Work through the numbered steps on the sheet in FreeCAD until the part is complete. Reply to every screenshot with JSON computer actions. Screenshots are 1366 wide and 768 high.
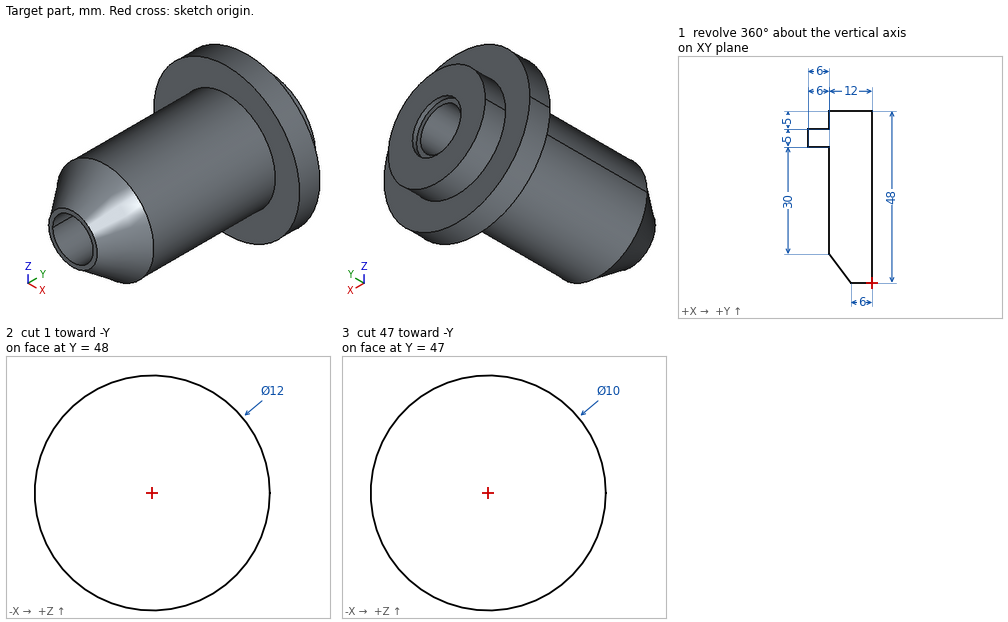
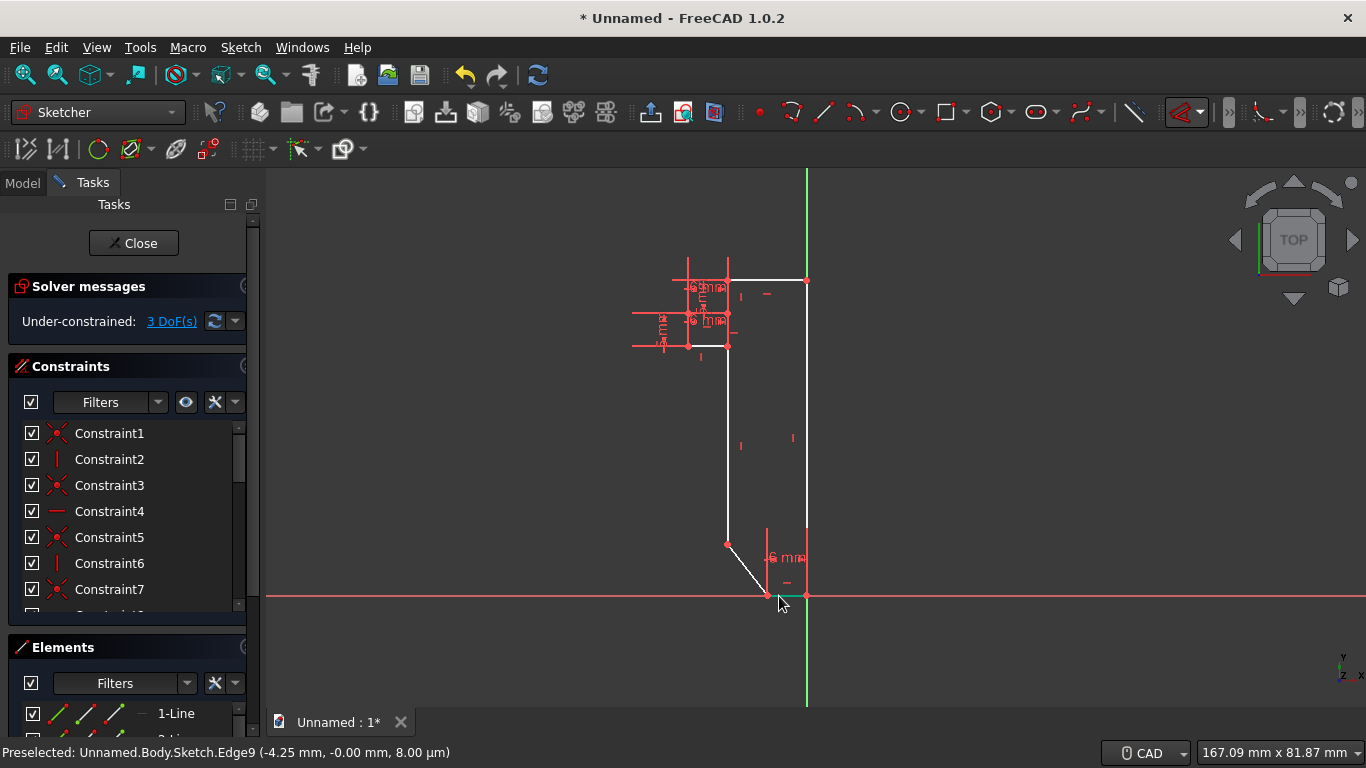
{"action": "left_click", "coordinate": [807, 501]}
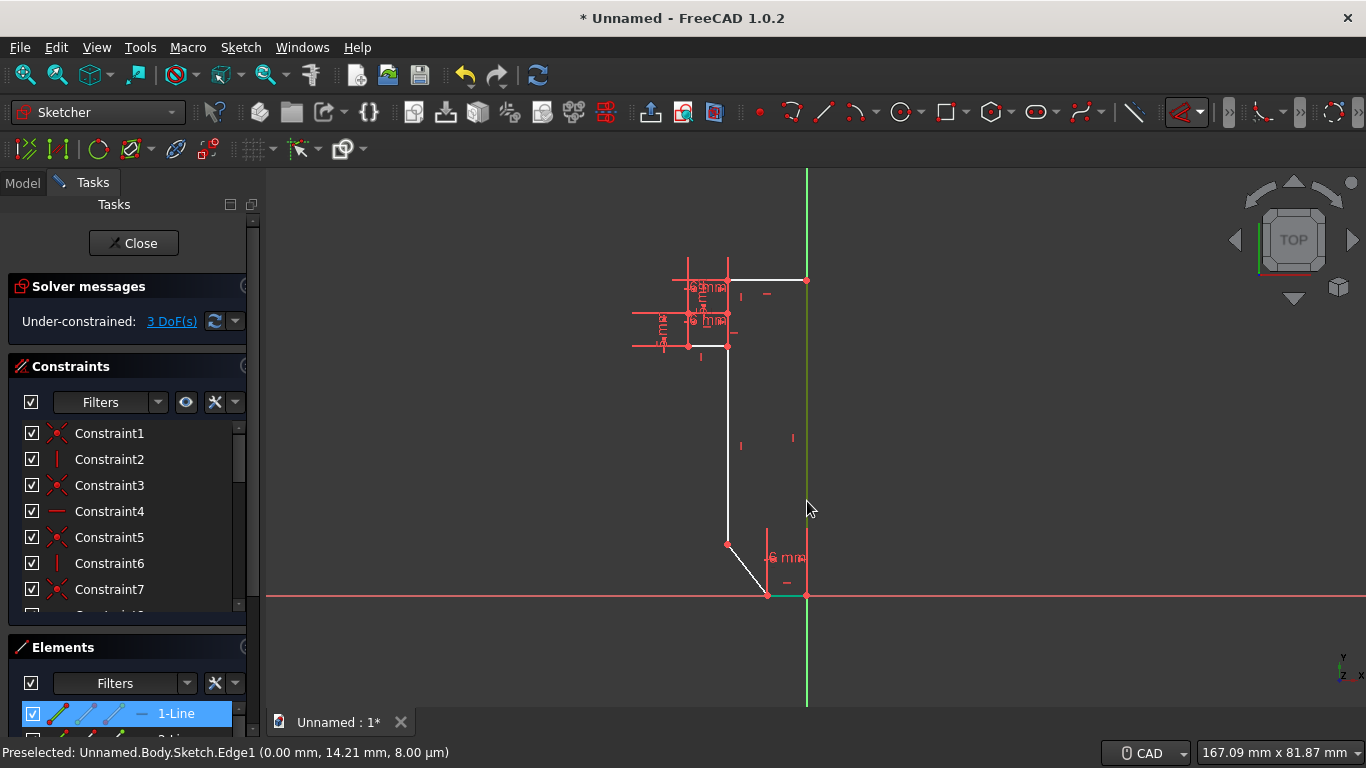
{"action": "key", "text": "i"}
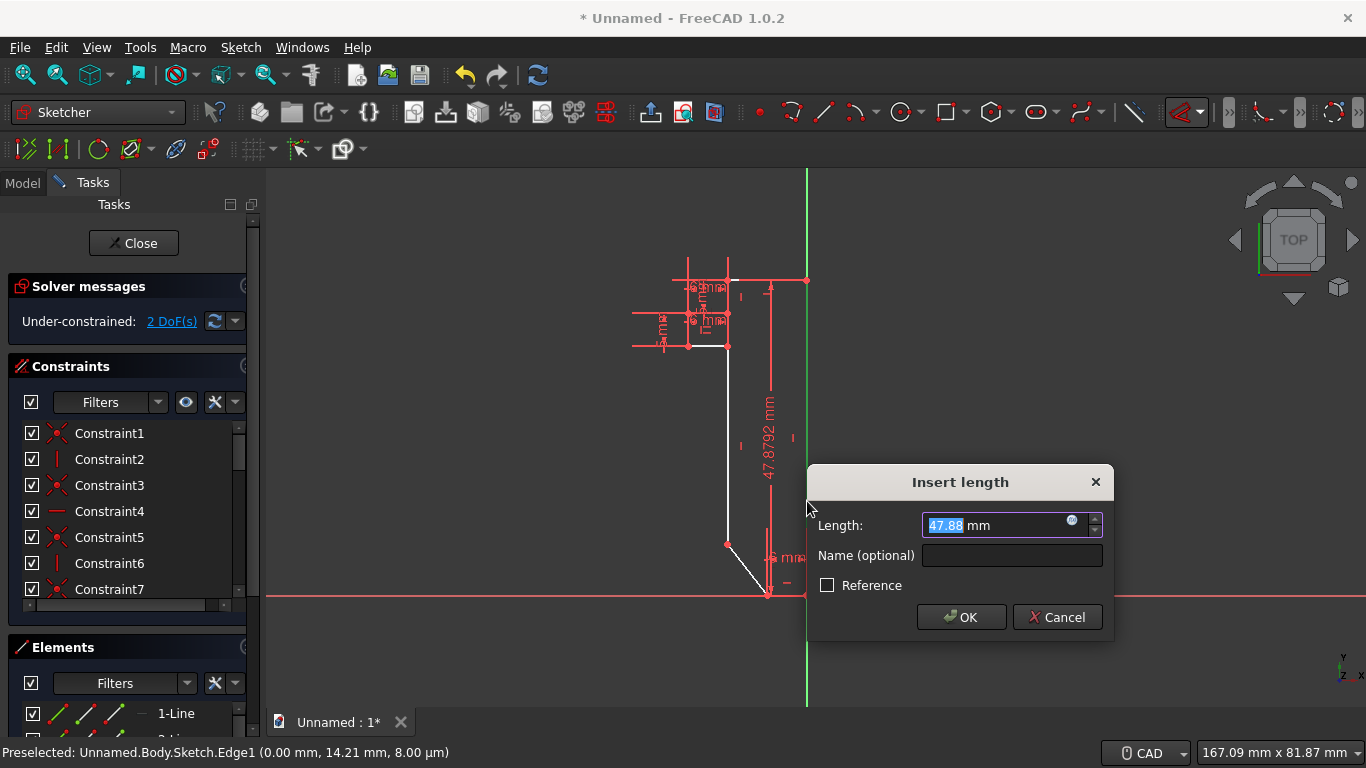
{"action": "type", "text": "48"}
{"action": "key", "text": "Return"}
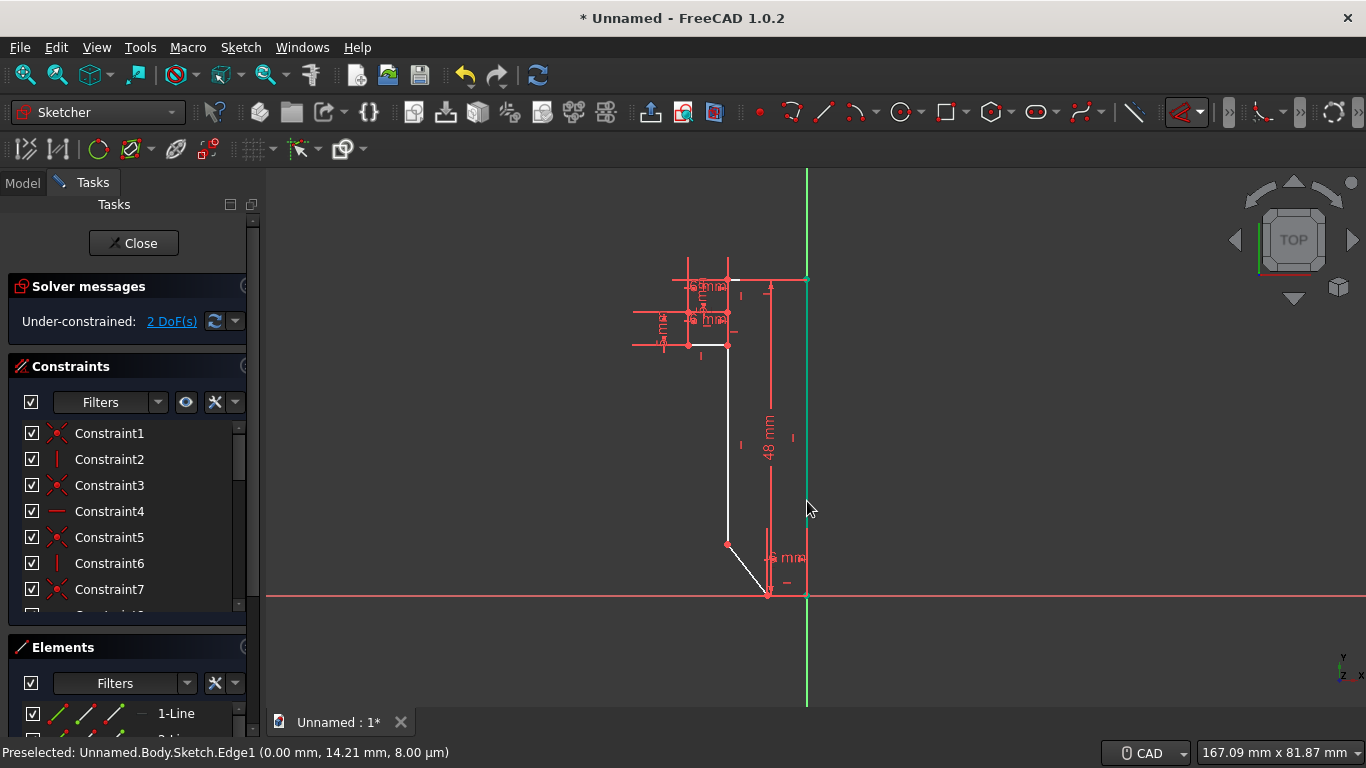
{"action": "left_click", "coordinate": [783, 280]}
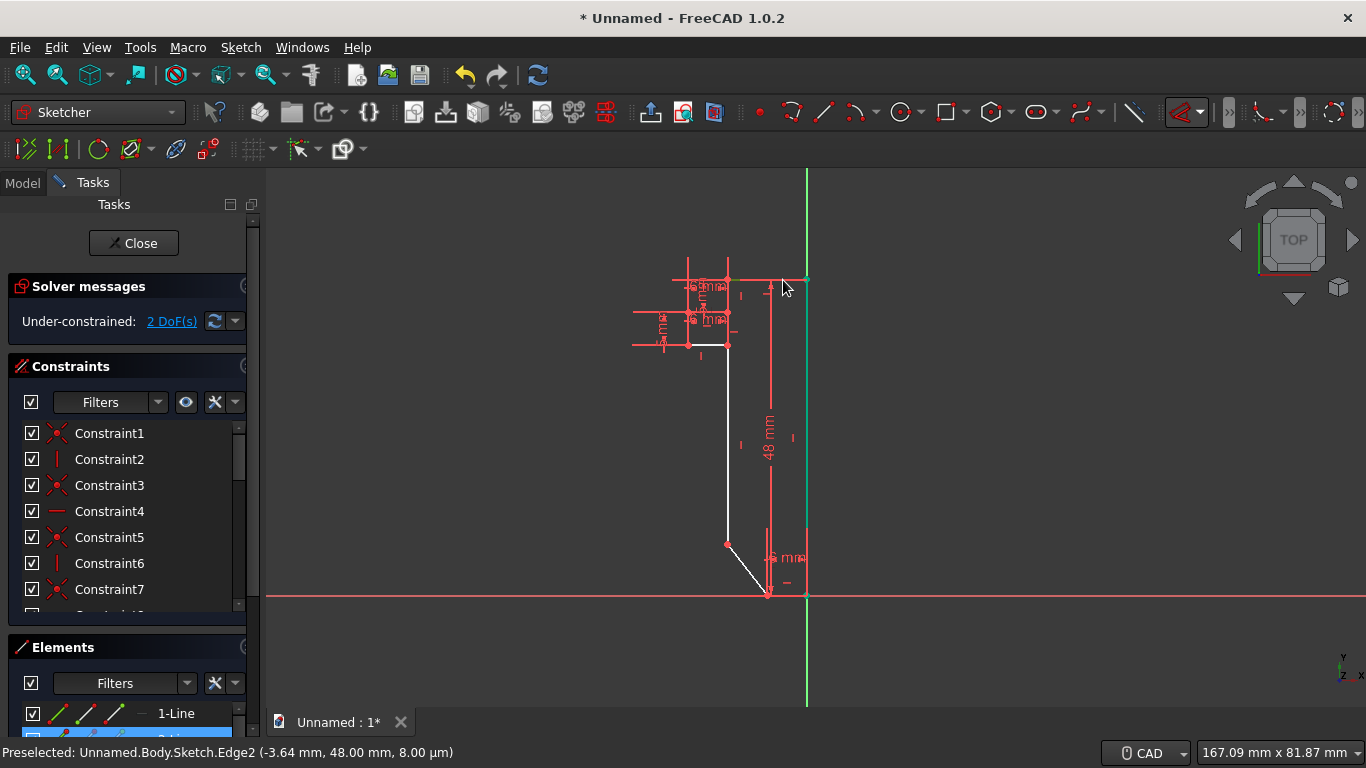
{"action": "left_click", "coordinate": [1202, 112]}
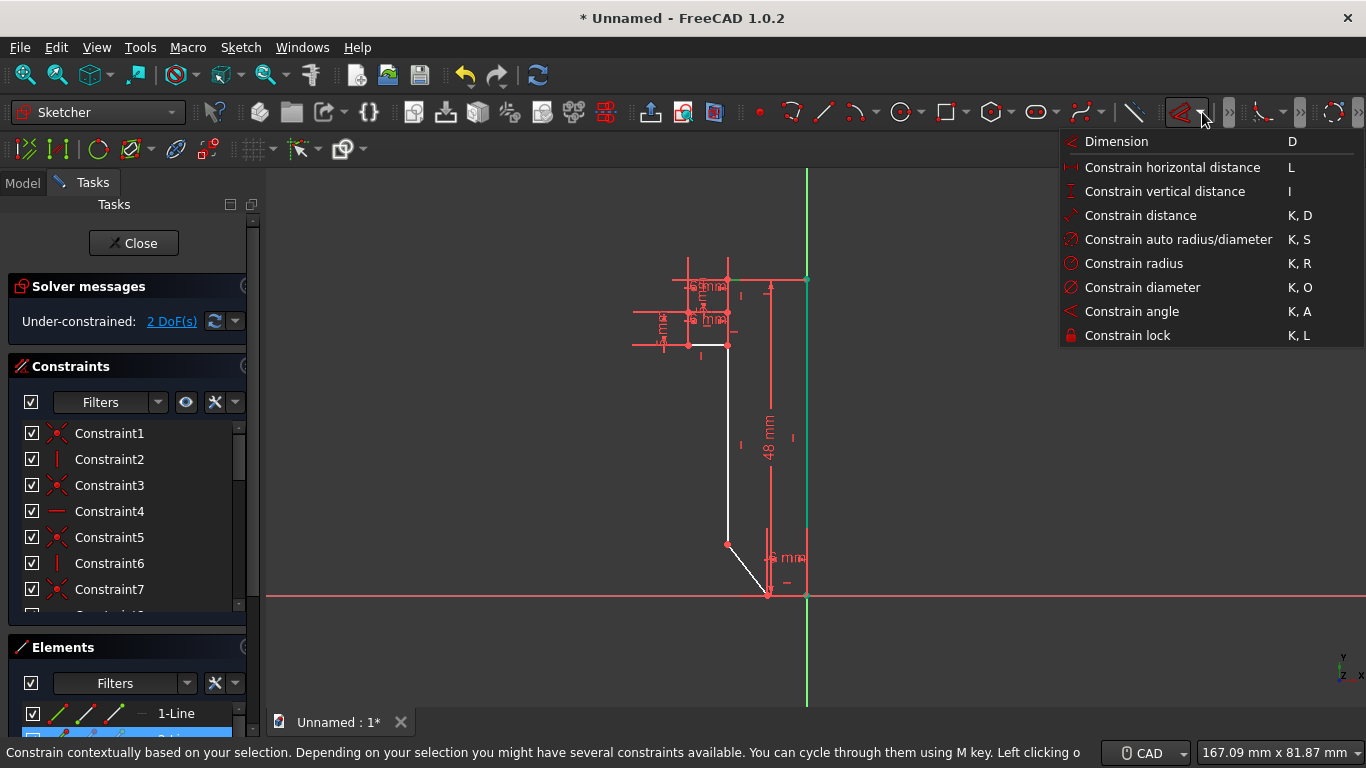
{"action": "left_click", "coordinate": [1212, 167]}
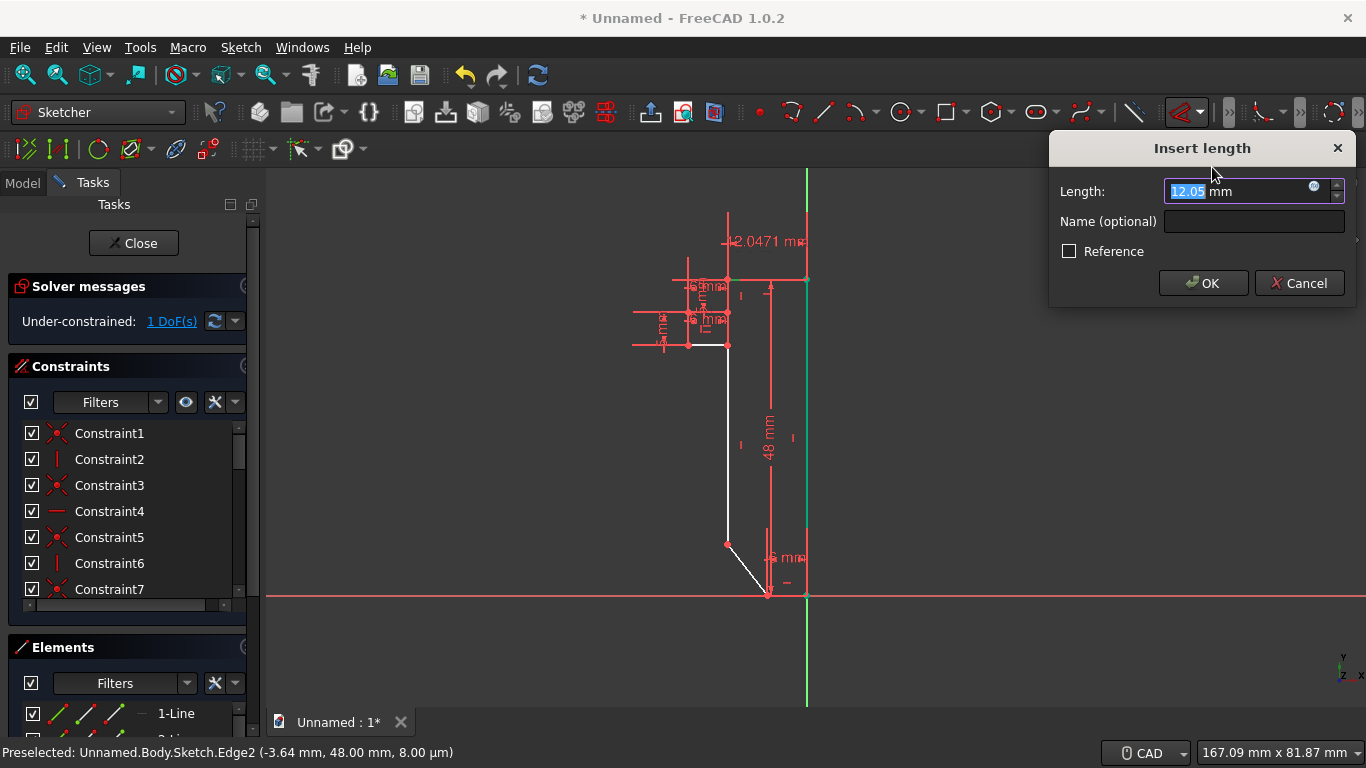
{"action": "type", "text": "12"}
{"action": "key", "text": "Return"}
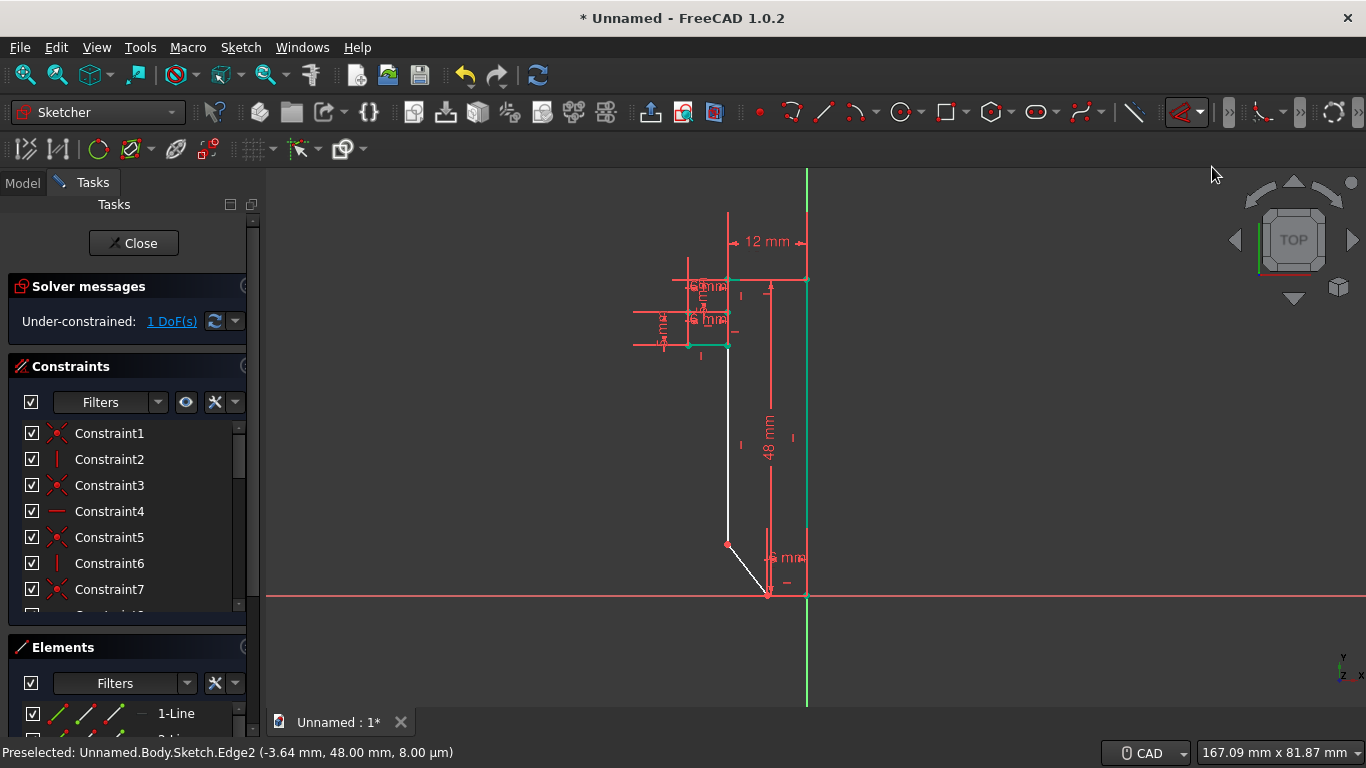
{"action": "left_click", "coordinate": [728, 405]}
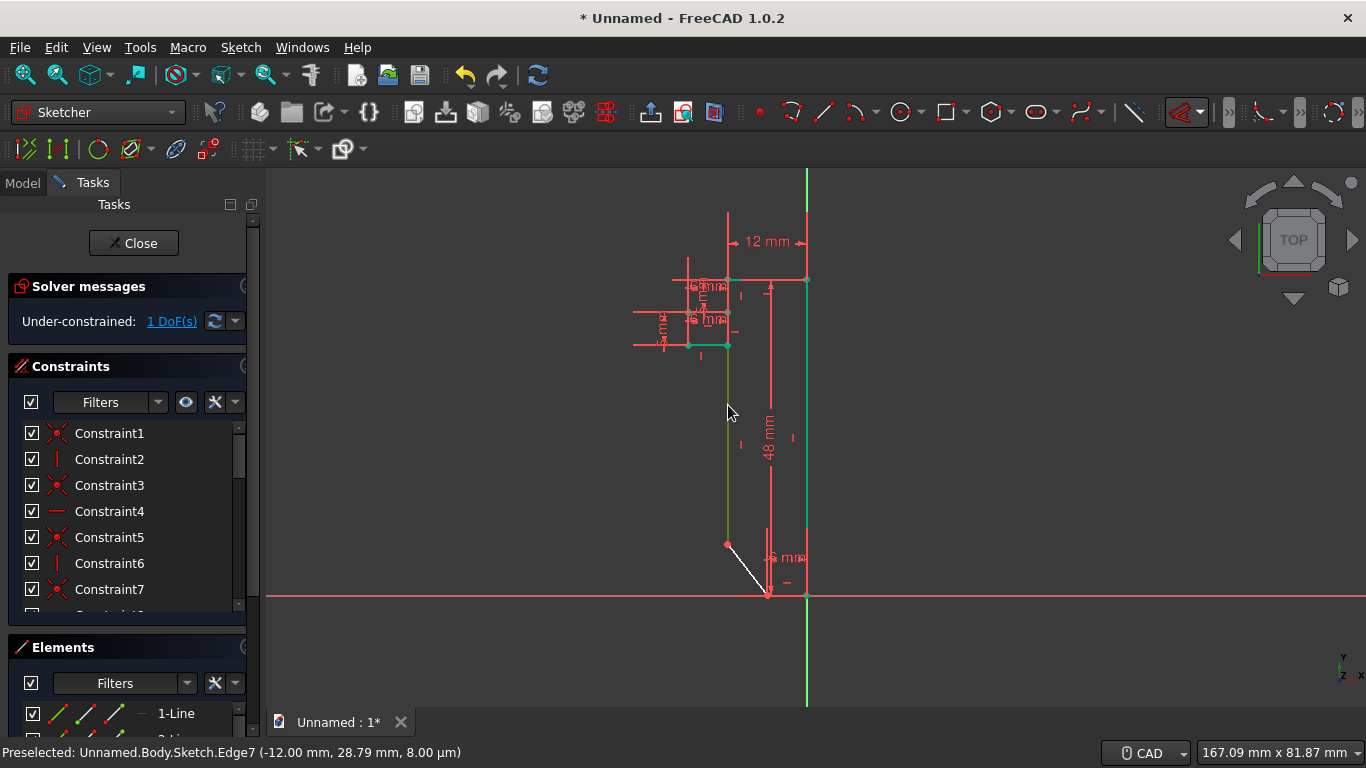
{"action": "left_click", "coordinate": [1202, 112]}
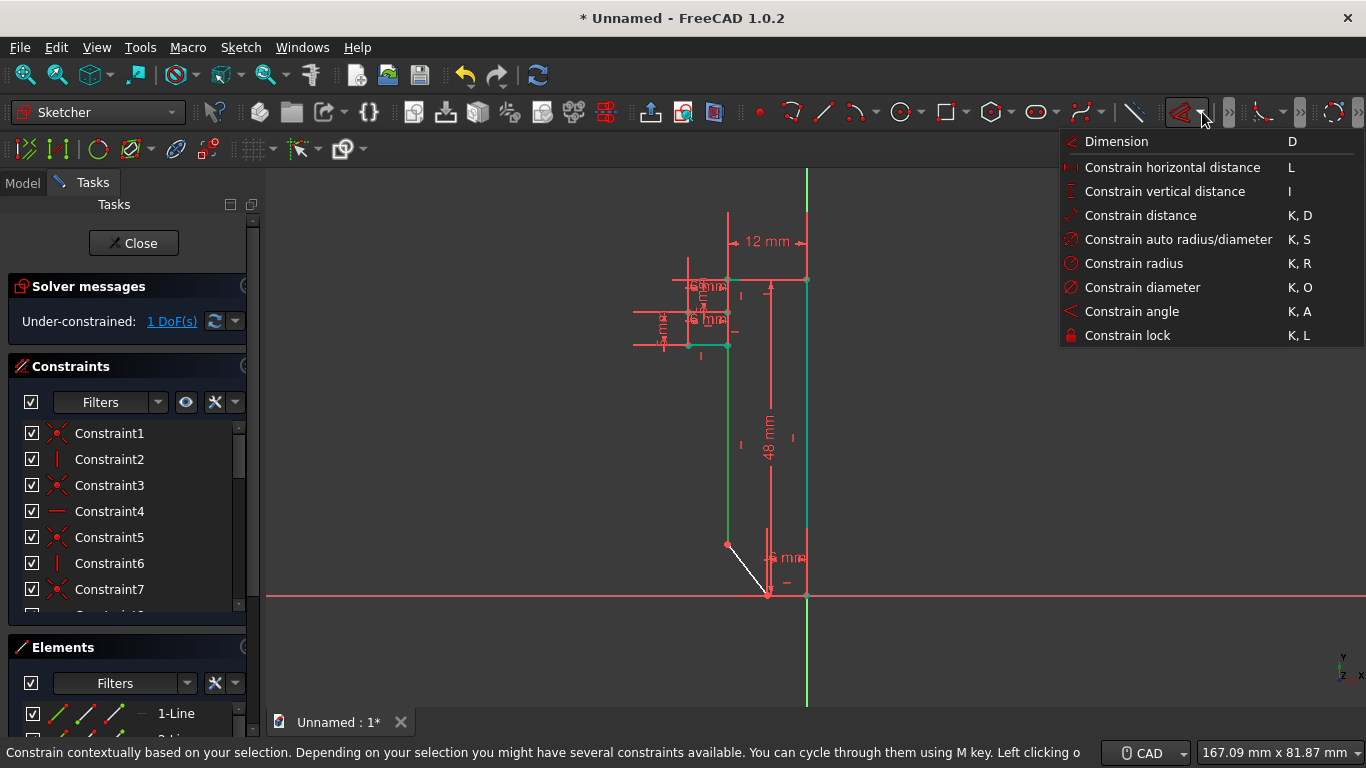
{"action": "left_click", "coordinate": [1212, 191]}